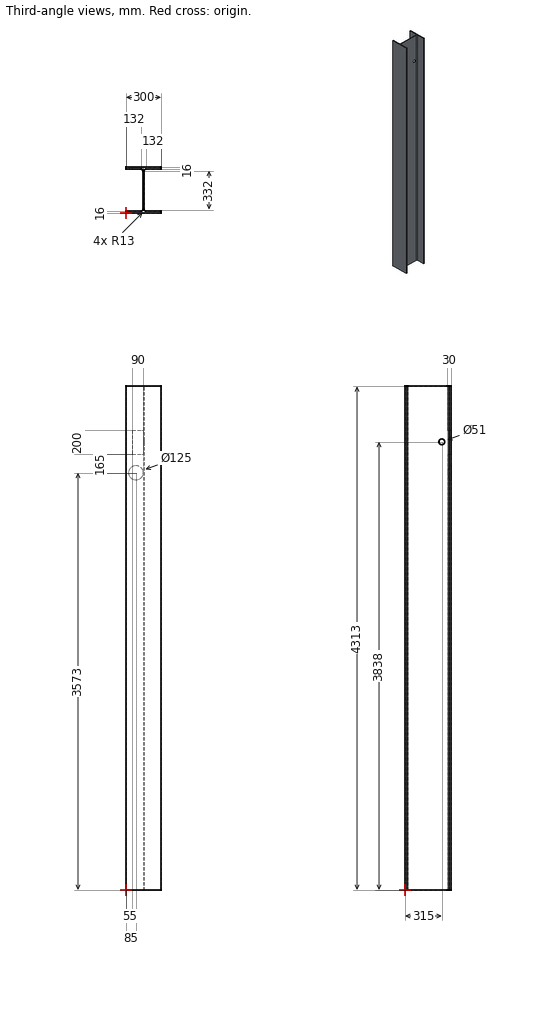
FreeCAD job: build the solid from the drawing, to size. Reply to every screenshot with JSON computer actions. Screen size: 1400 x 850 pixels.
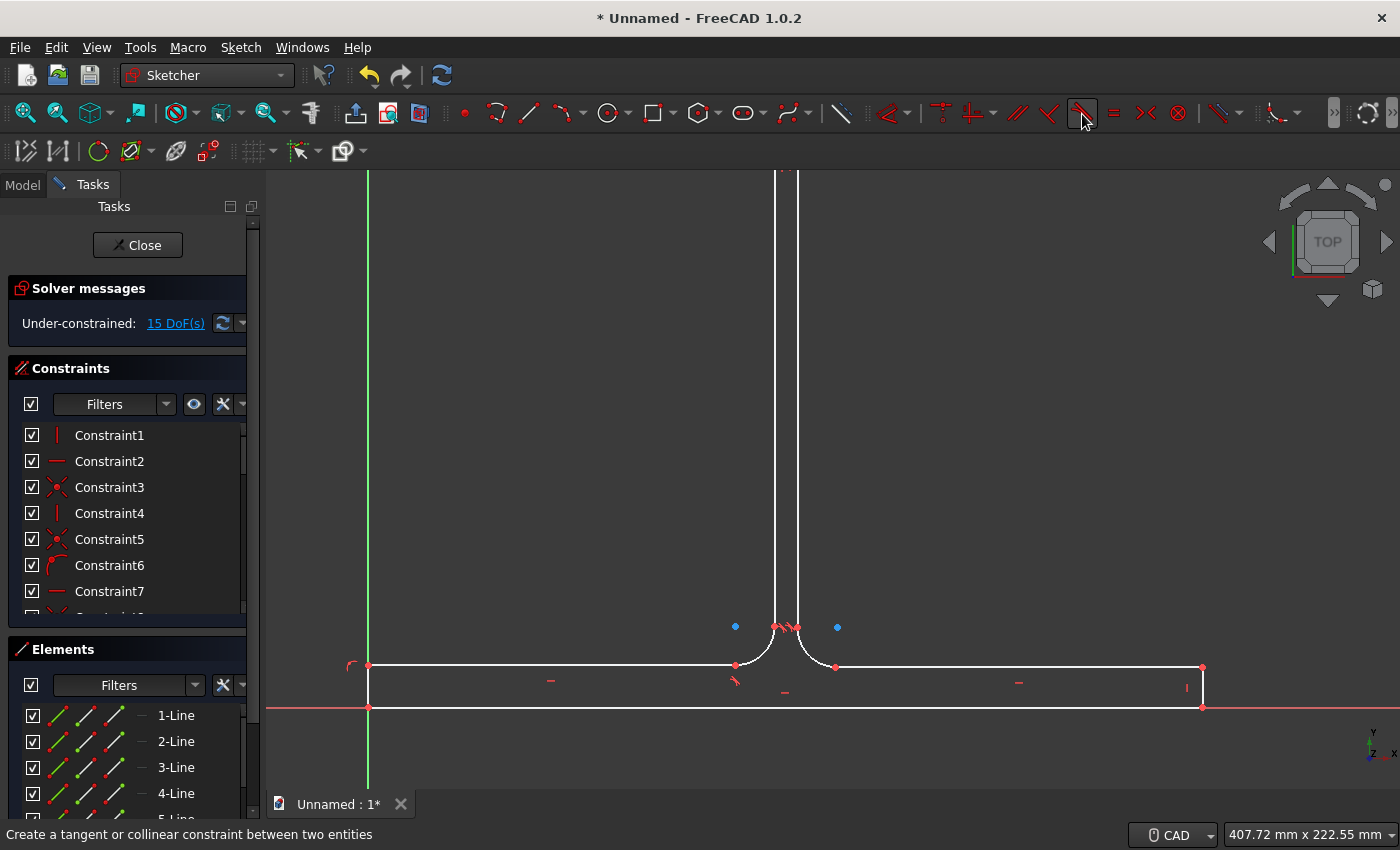
{"action": "left_click", "coordinate": [1093, 667]}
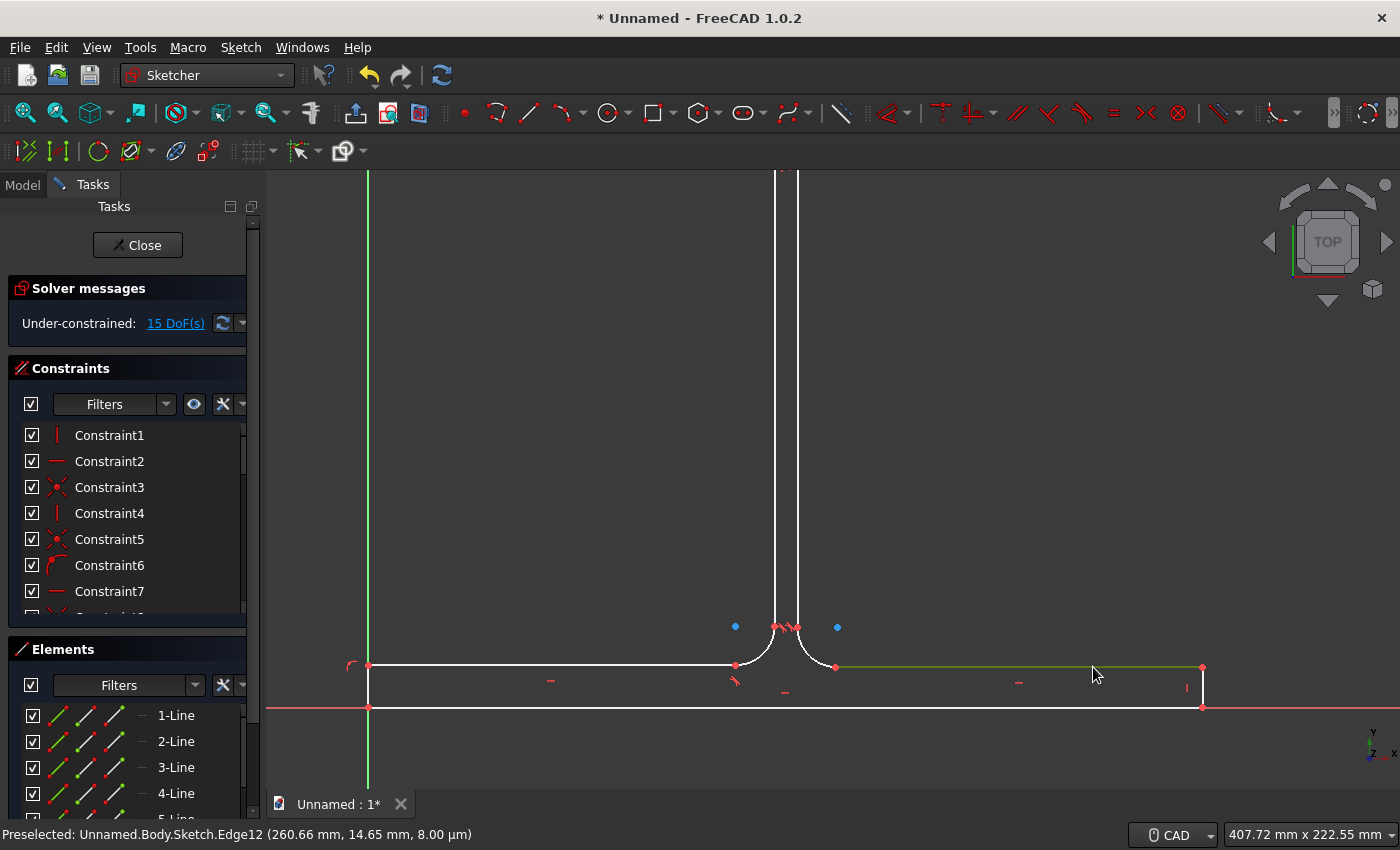
{"action": "left_click", "coordinate": [802, 645]}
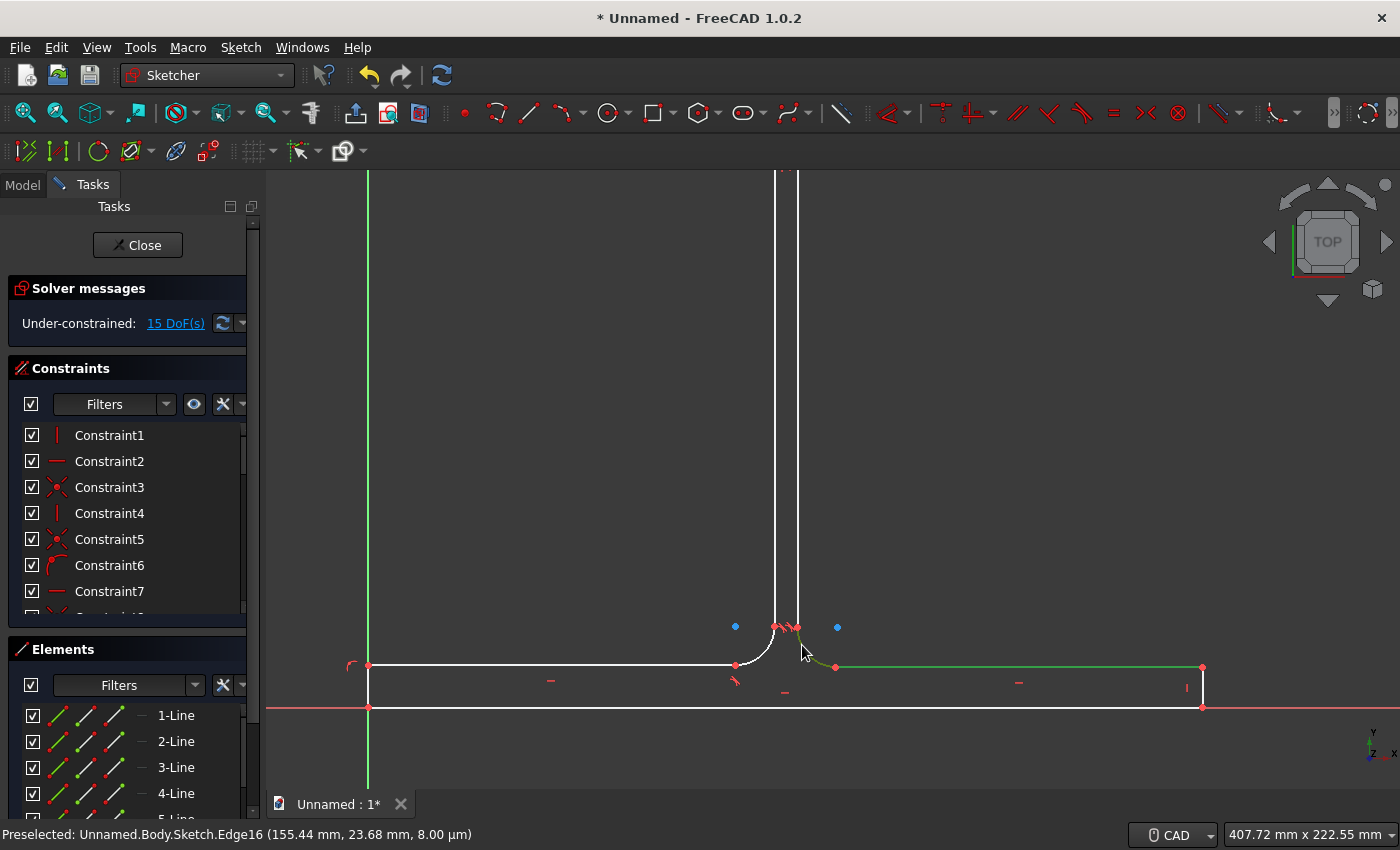
{"action": "left_click", "coordinate": [1082, 114]}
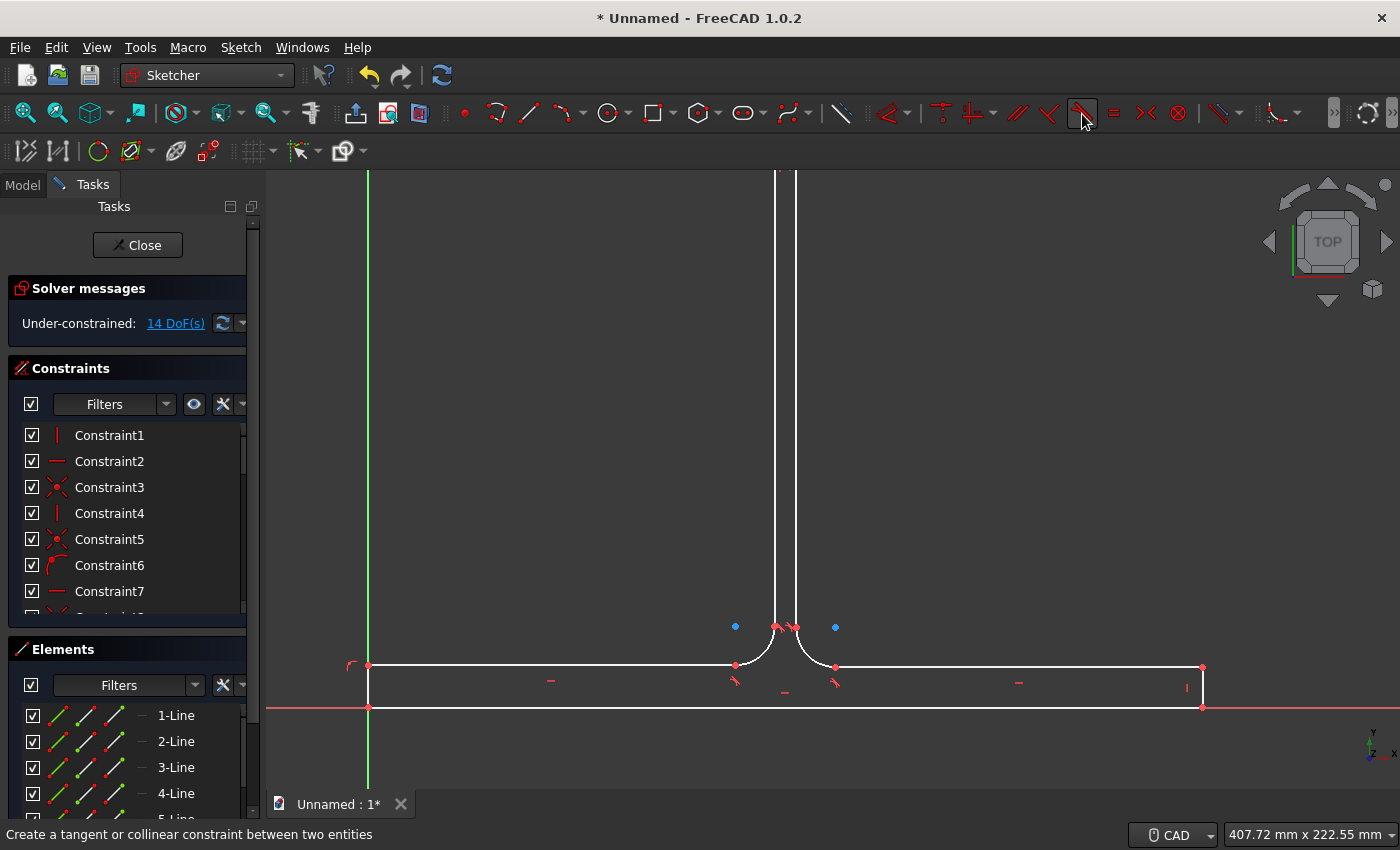
{"action": "scroll", "coordinate": [752, 662], "scroll_direction": "down", "scroll_amount": 5}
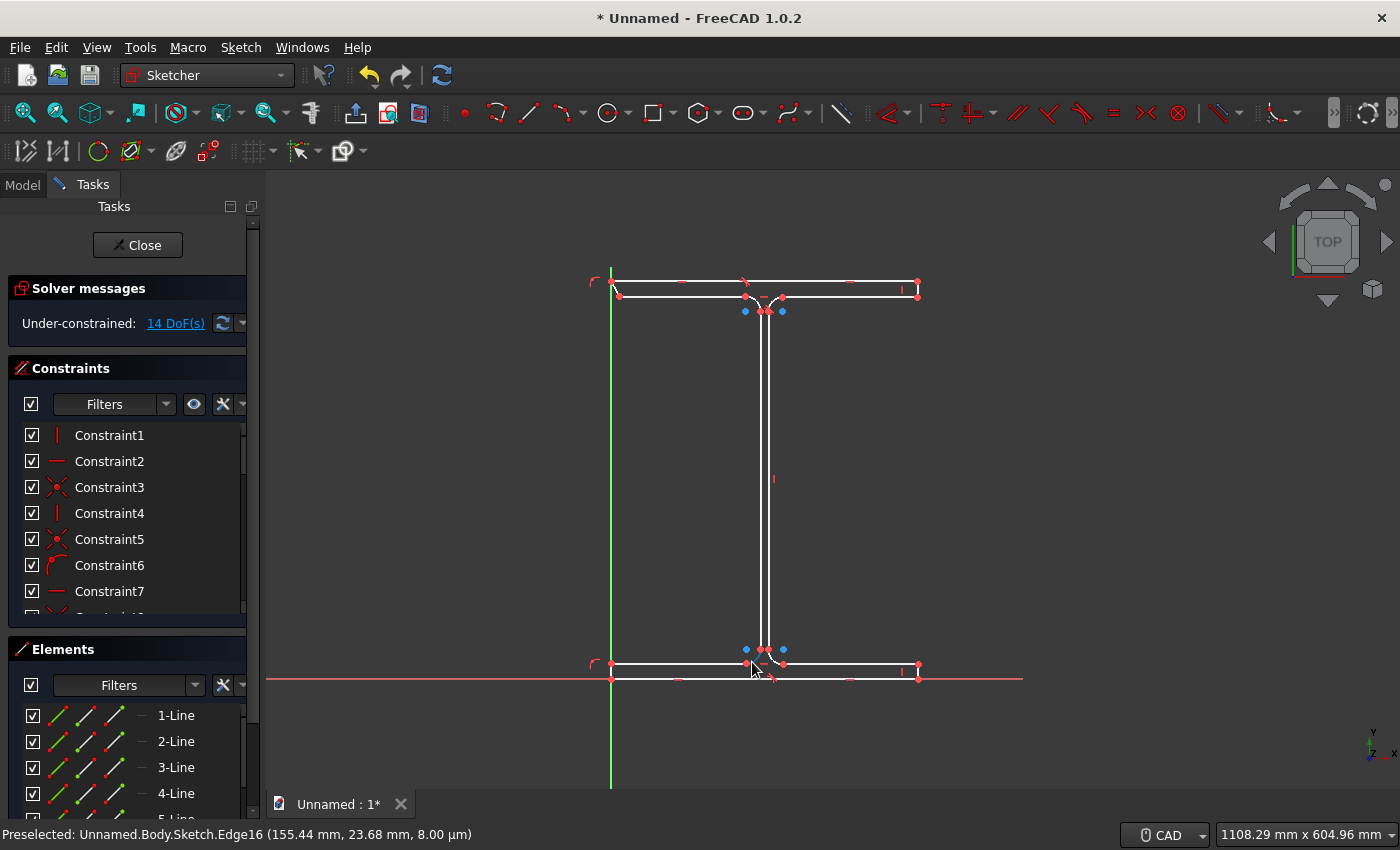
{"action": "scroll", "coordinate": [617, 292], "scroll_direction": "up", "scroll_amount": 5}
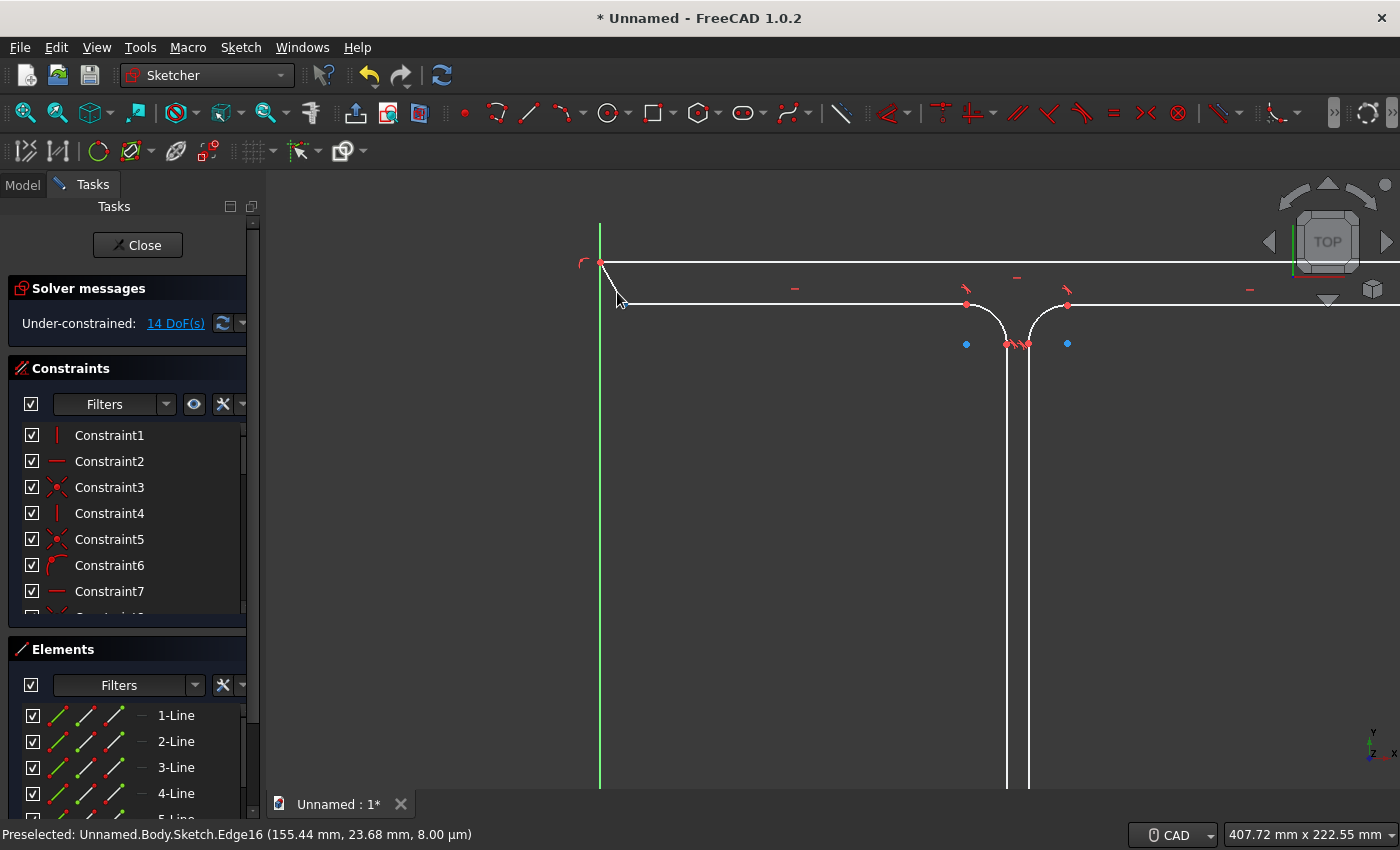
{"action": "left_click", "coordinate": [617, 292]}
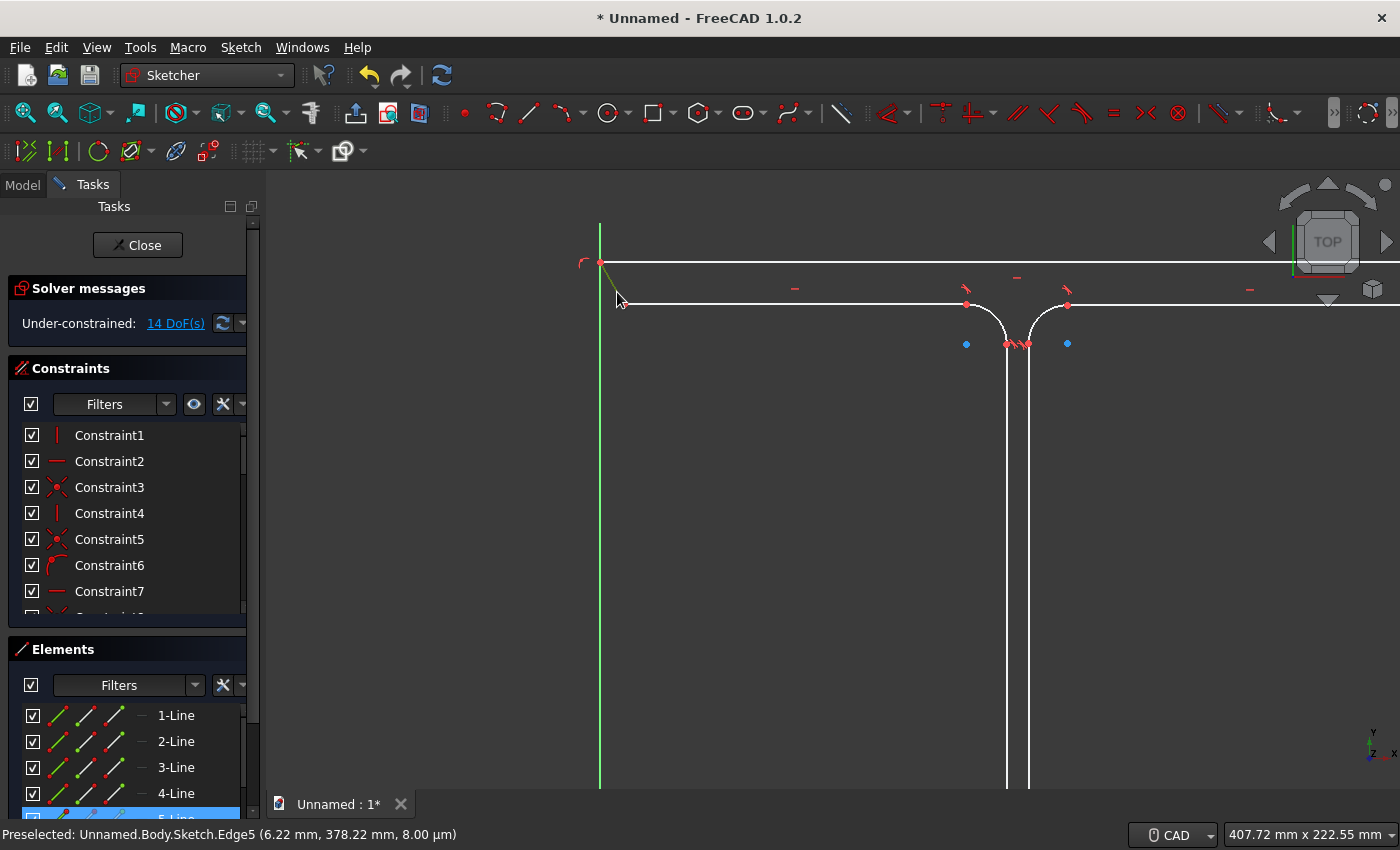
{"action": "key", "text": "v"}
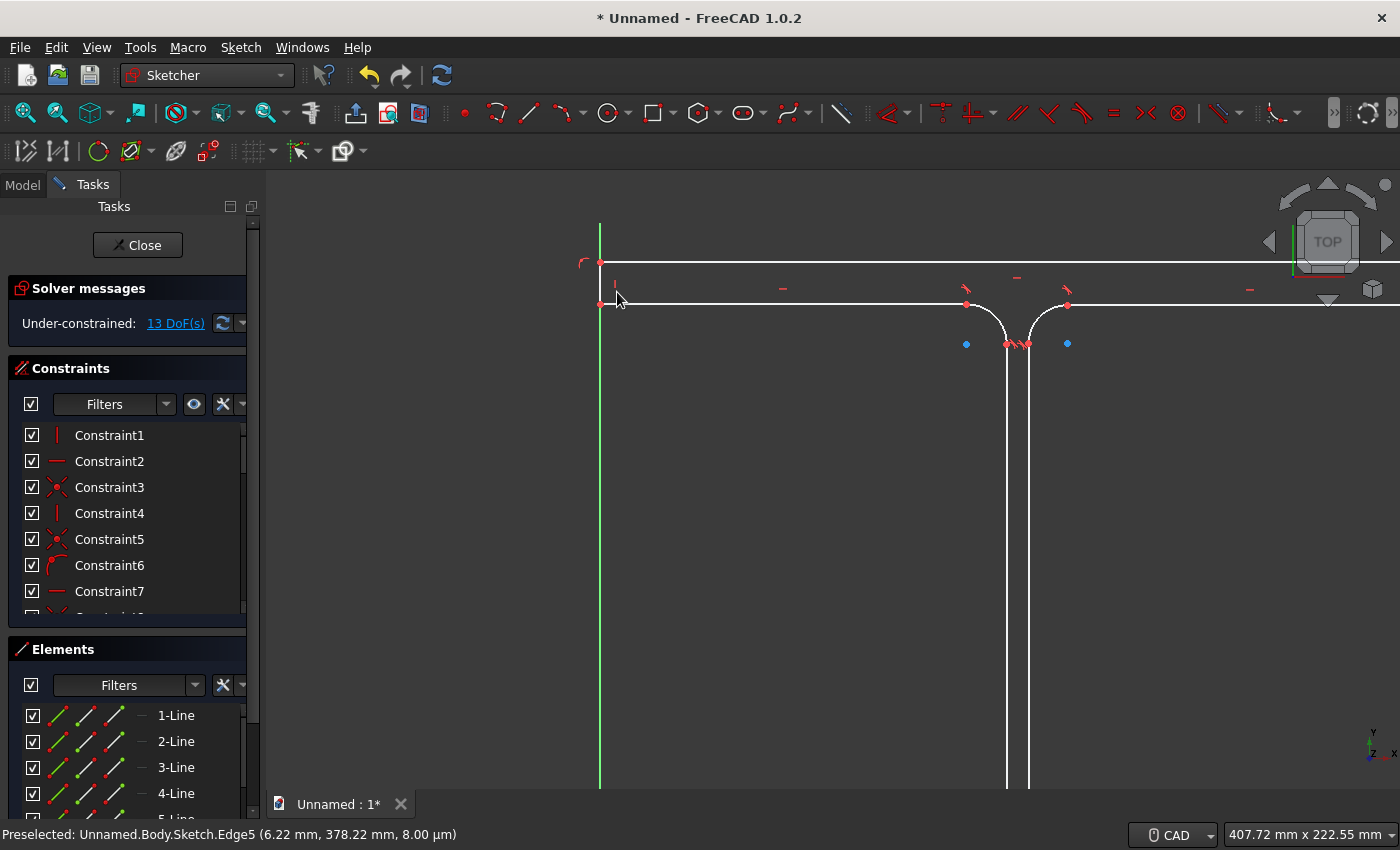
{"action": "left_click", "coordinate": [1050, 310]}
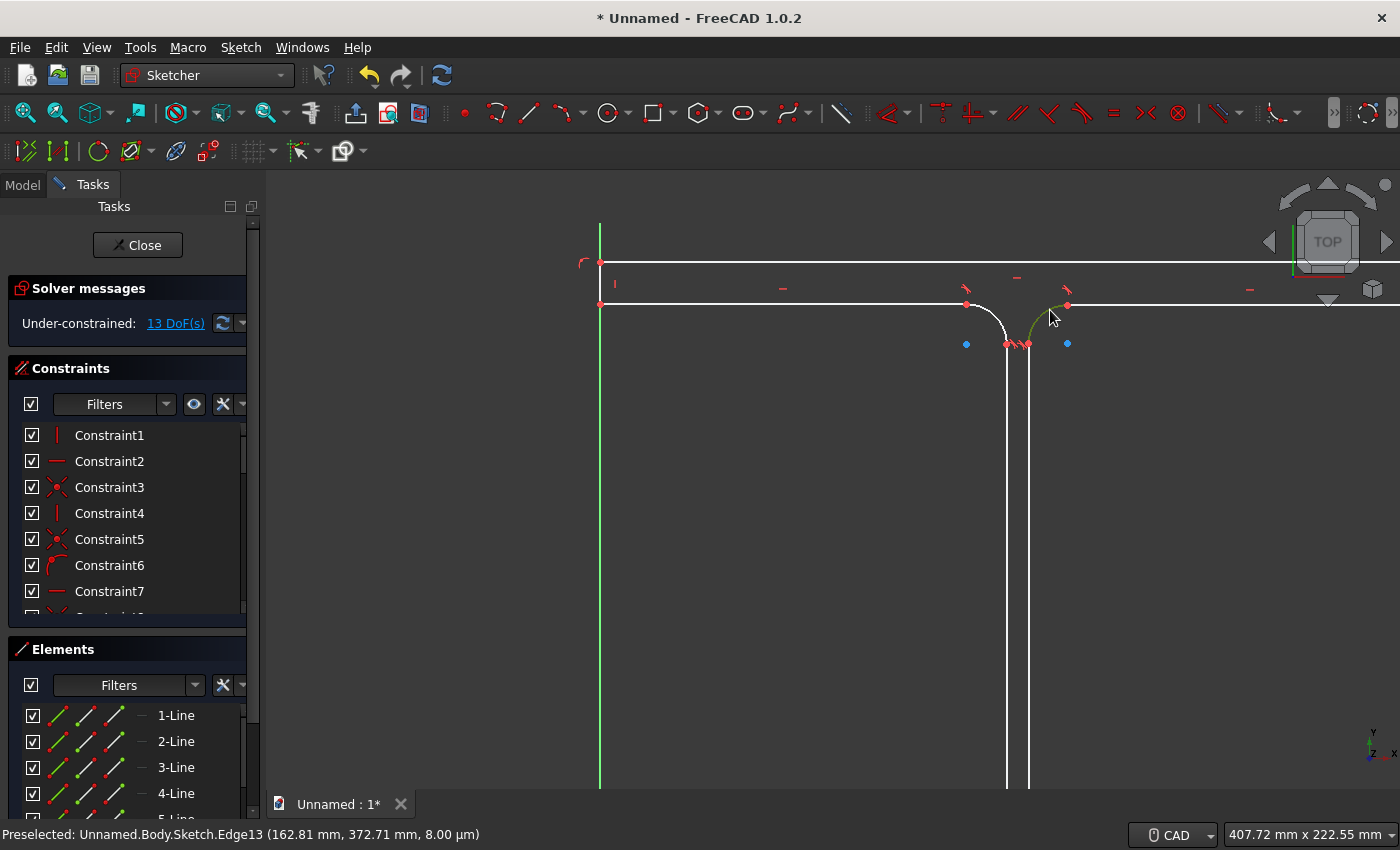
{"action": "left_click", "coordinate": [1002, 326]}